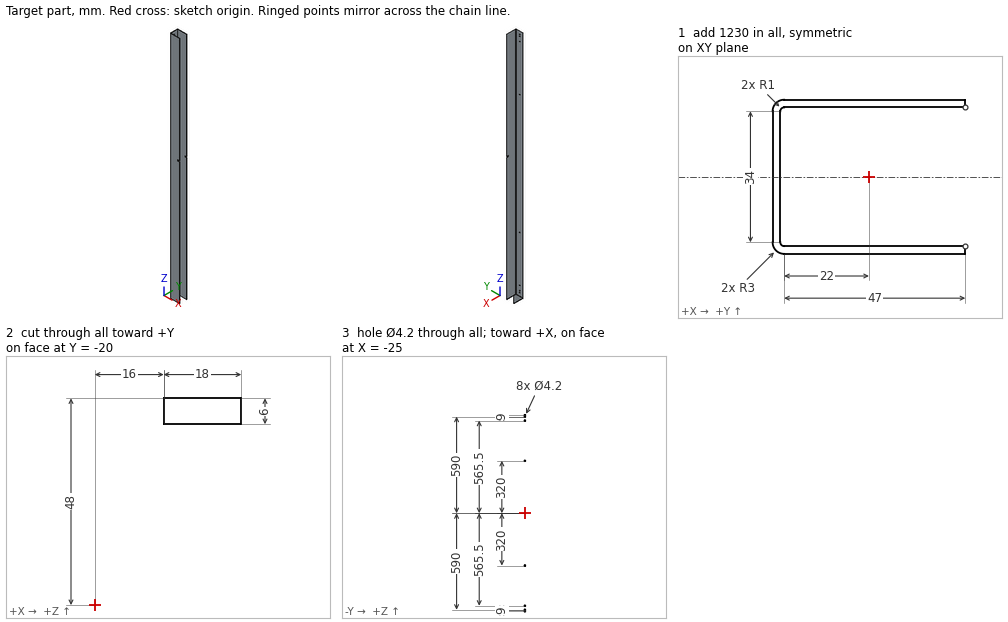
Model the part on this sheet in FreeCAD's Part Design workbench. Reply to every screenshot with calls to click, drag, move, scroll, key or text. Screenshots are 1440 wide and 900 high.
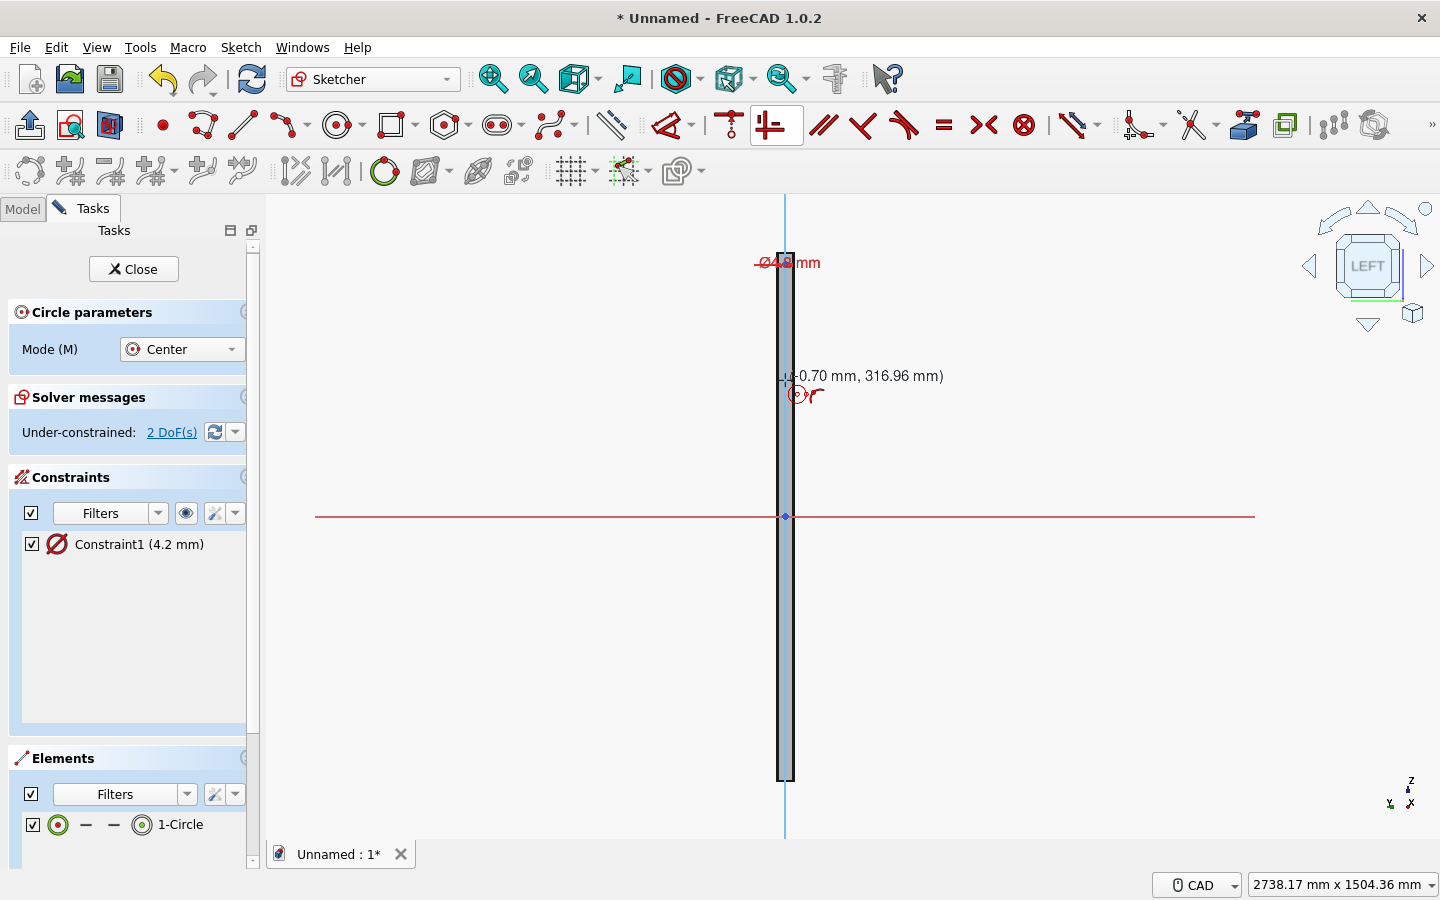
click(785, 380)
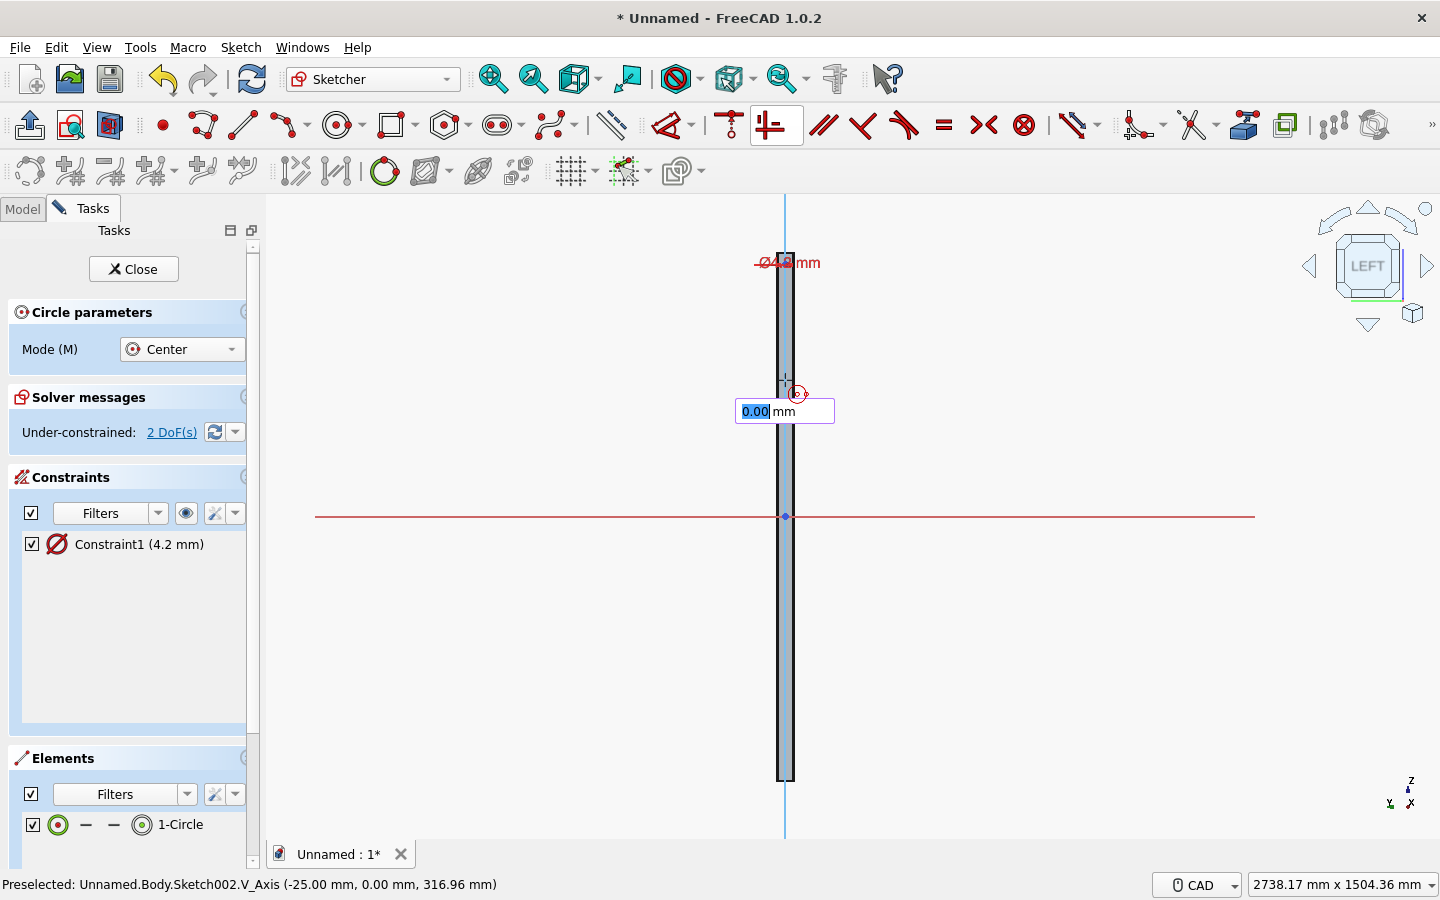
scroll(786, 379, up, 15)
move(780, 381)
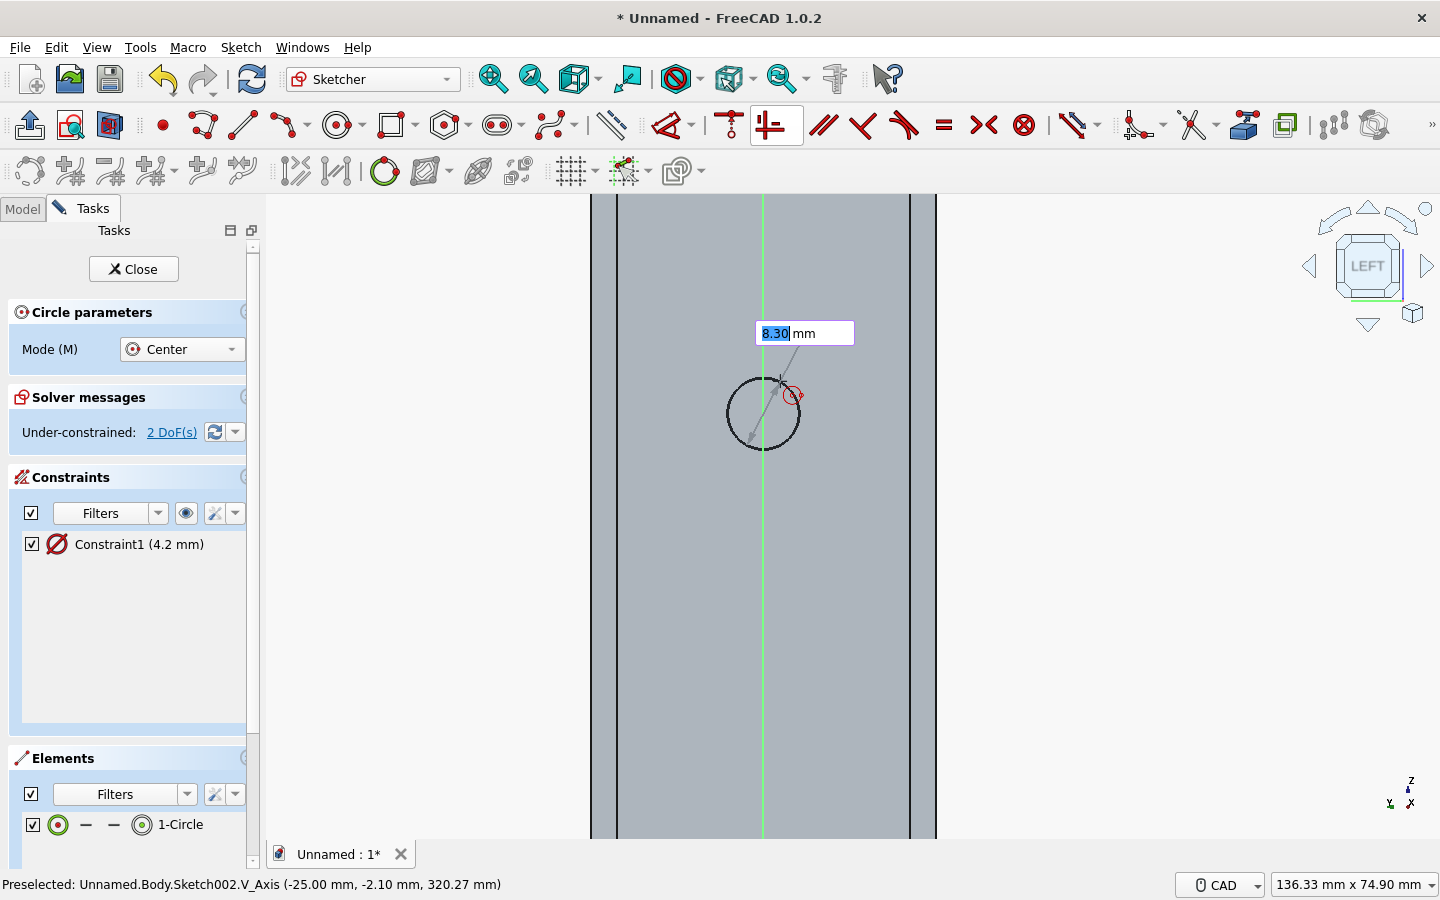
text(4.2)
key(Return)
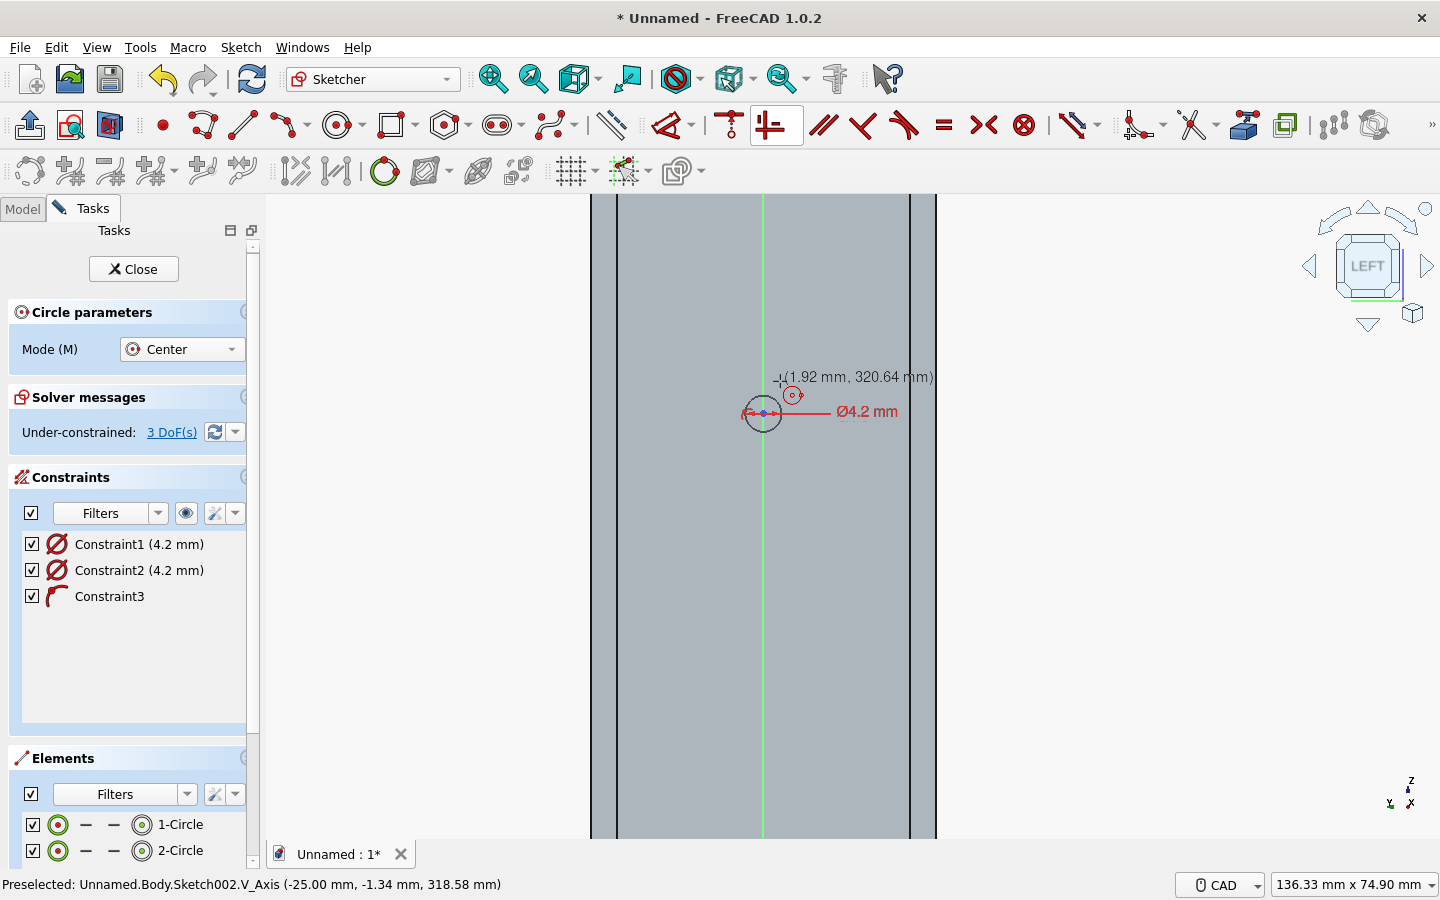
scroll(786, 379, down, 15)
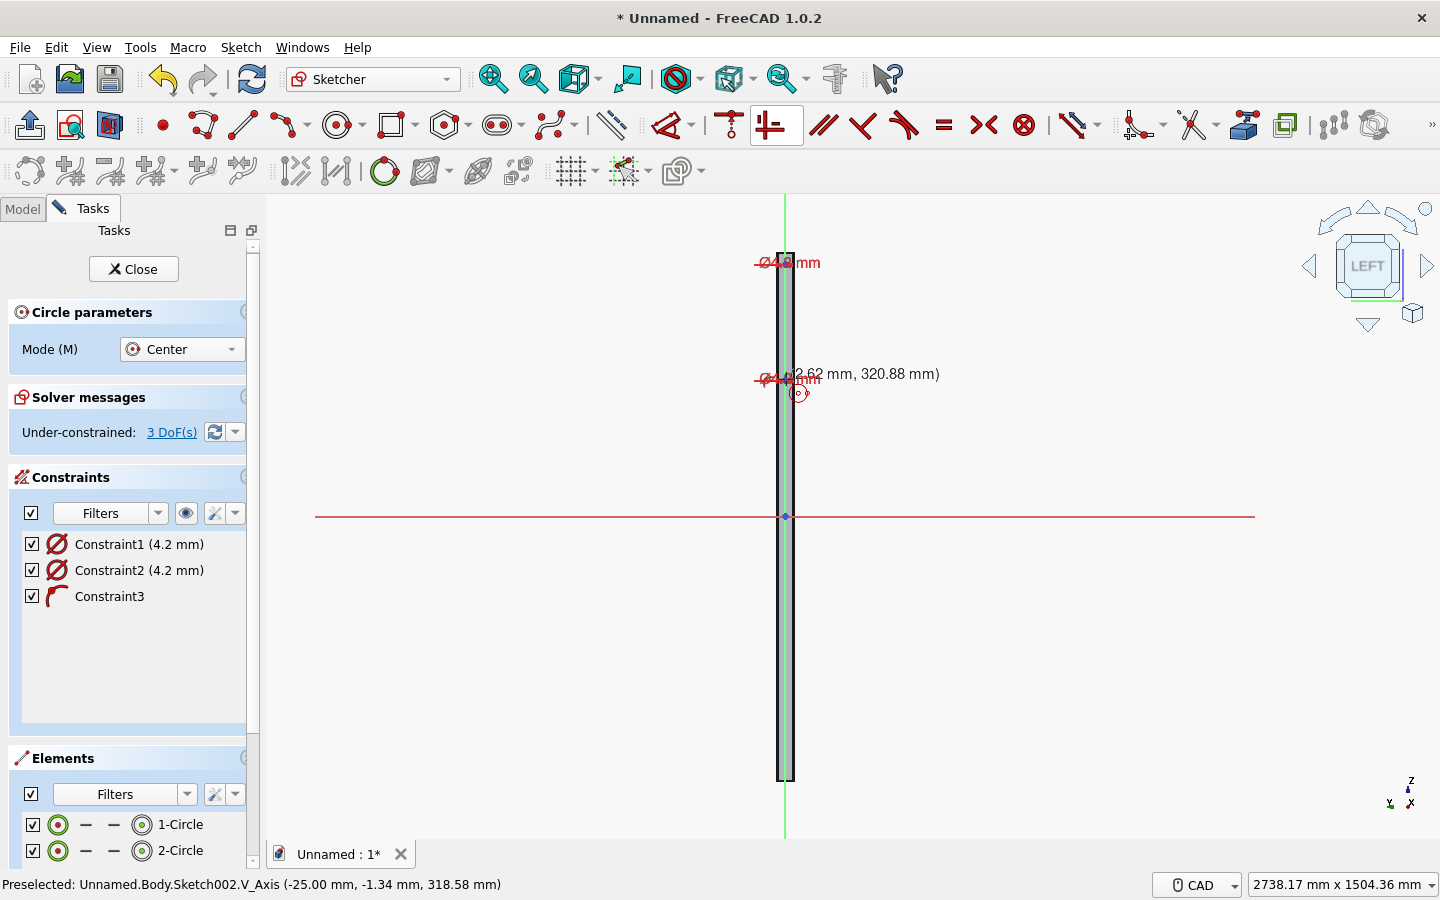
scroll(785, 654, up, 17)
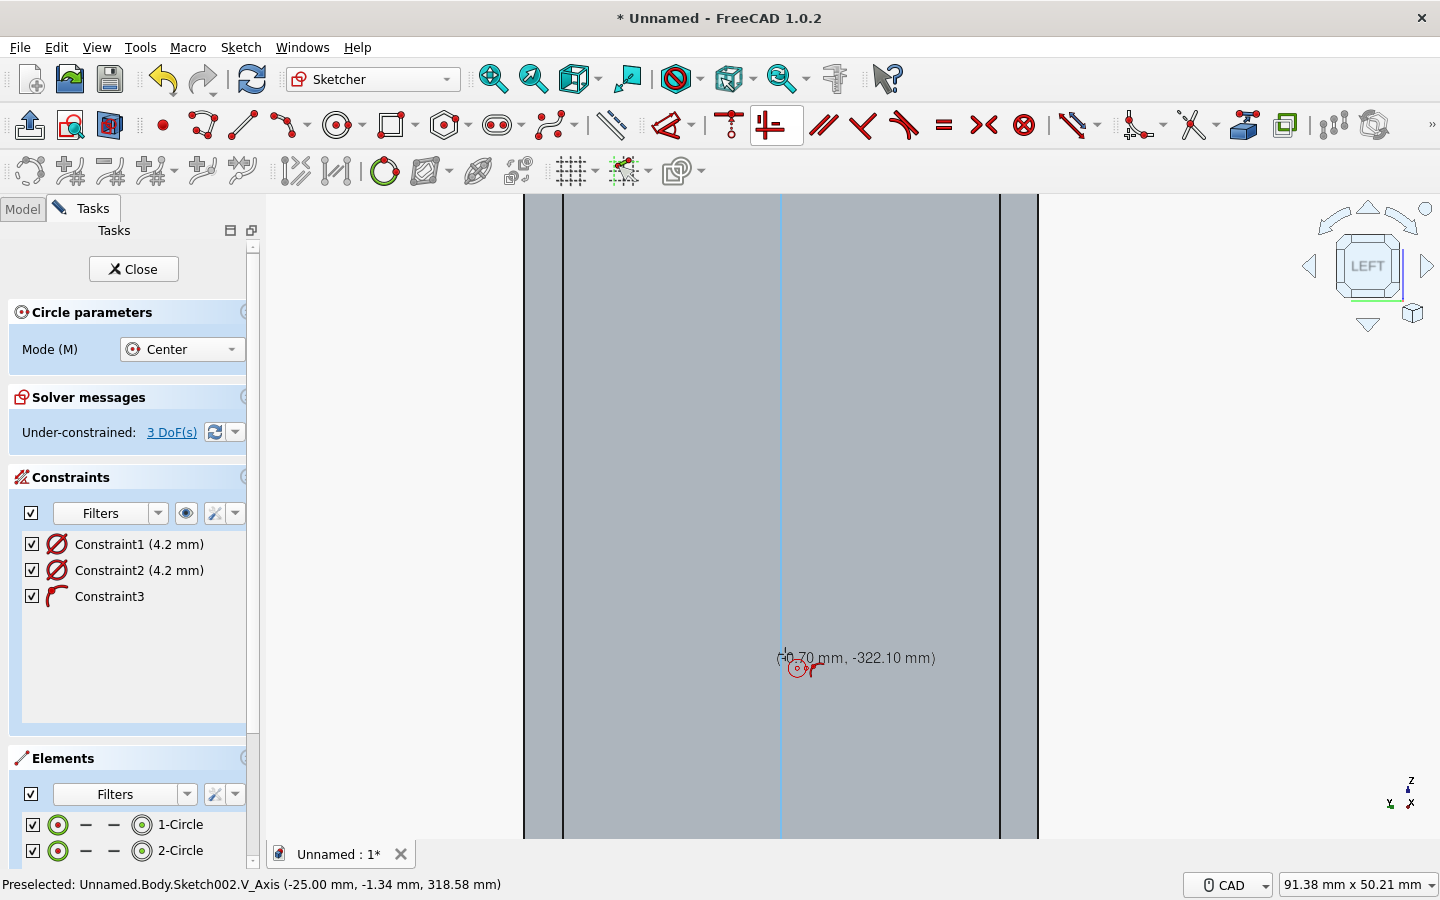
scroll(785, 654, down, 17)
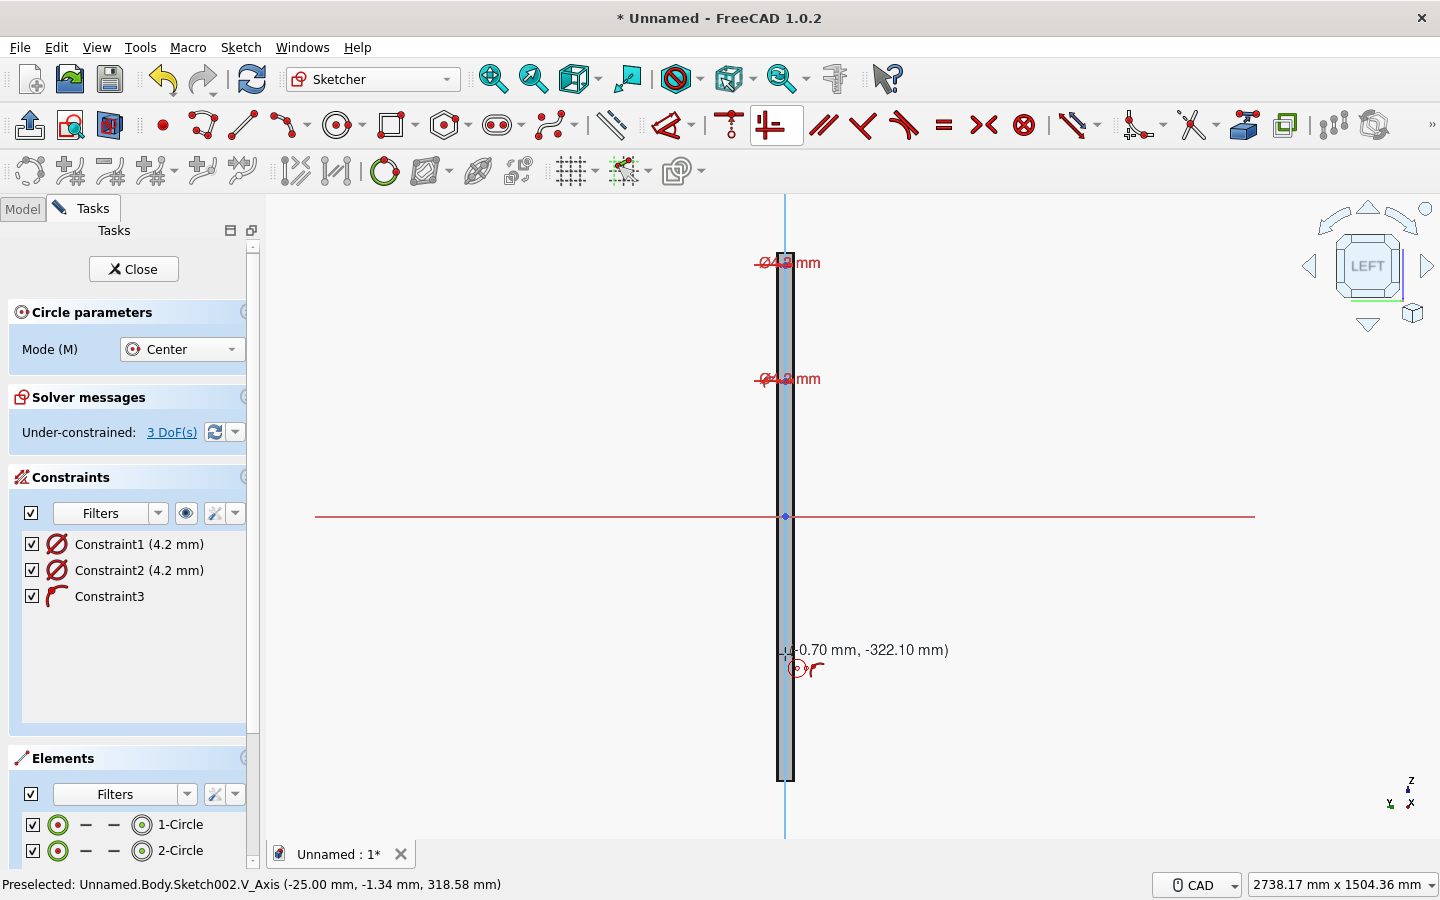
click(785, 654)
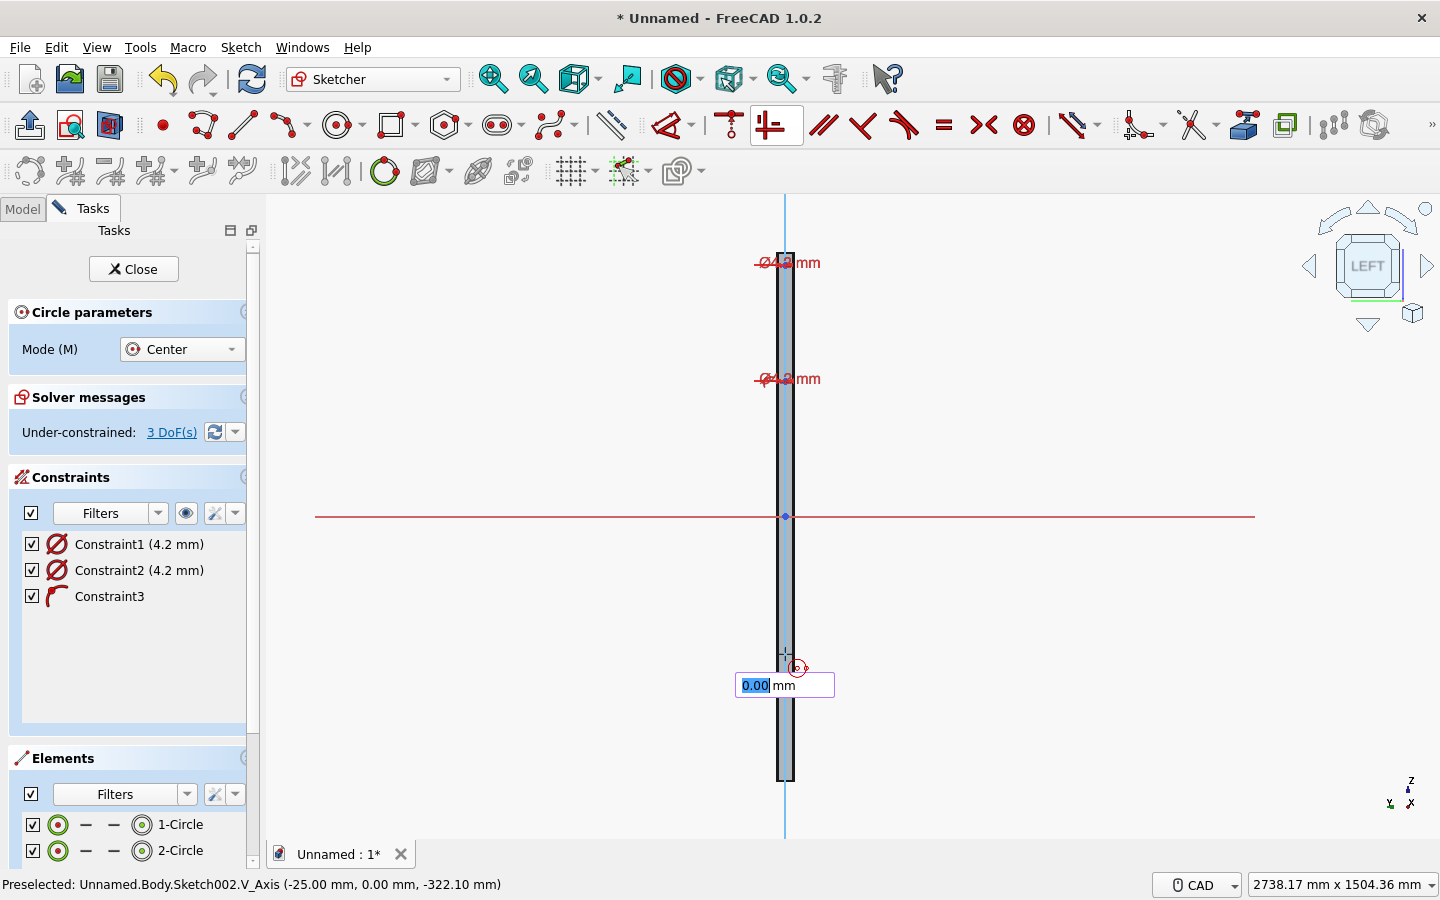
scroll(786, 654, up, 15)
move(780, 636)